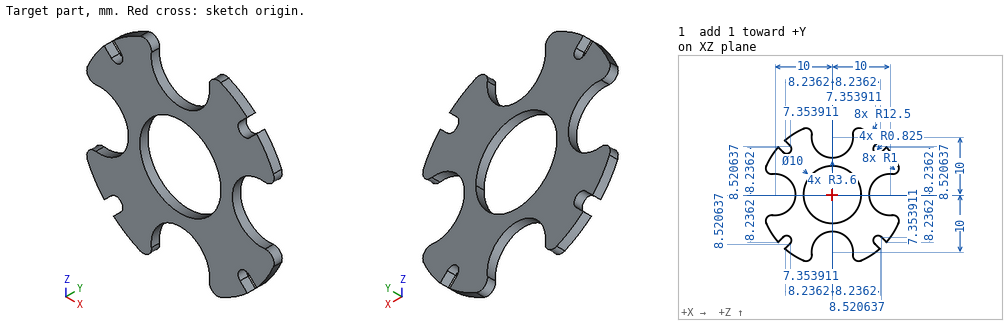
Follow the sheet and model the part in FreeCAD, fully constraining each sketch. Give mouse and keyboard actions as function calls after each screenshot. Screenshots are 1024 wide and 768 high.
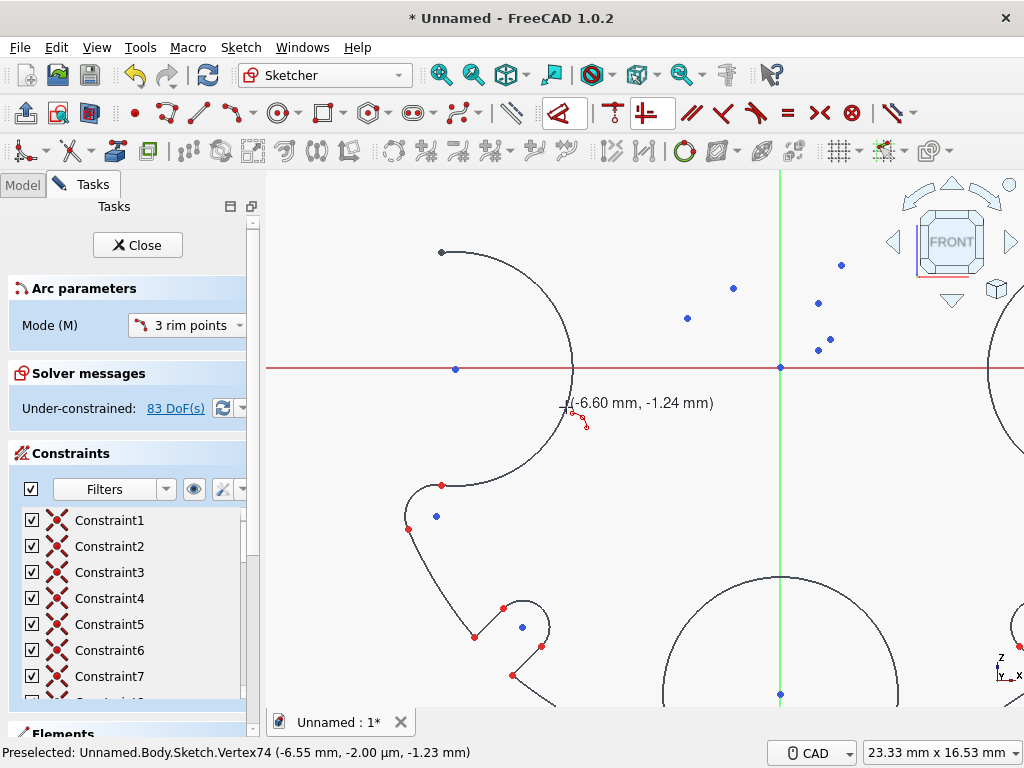
click(441, 253)
click(408, 206)
click(411, 239)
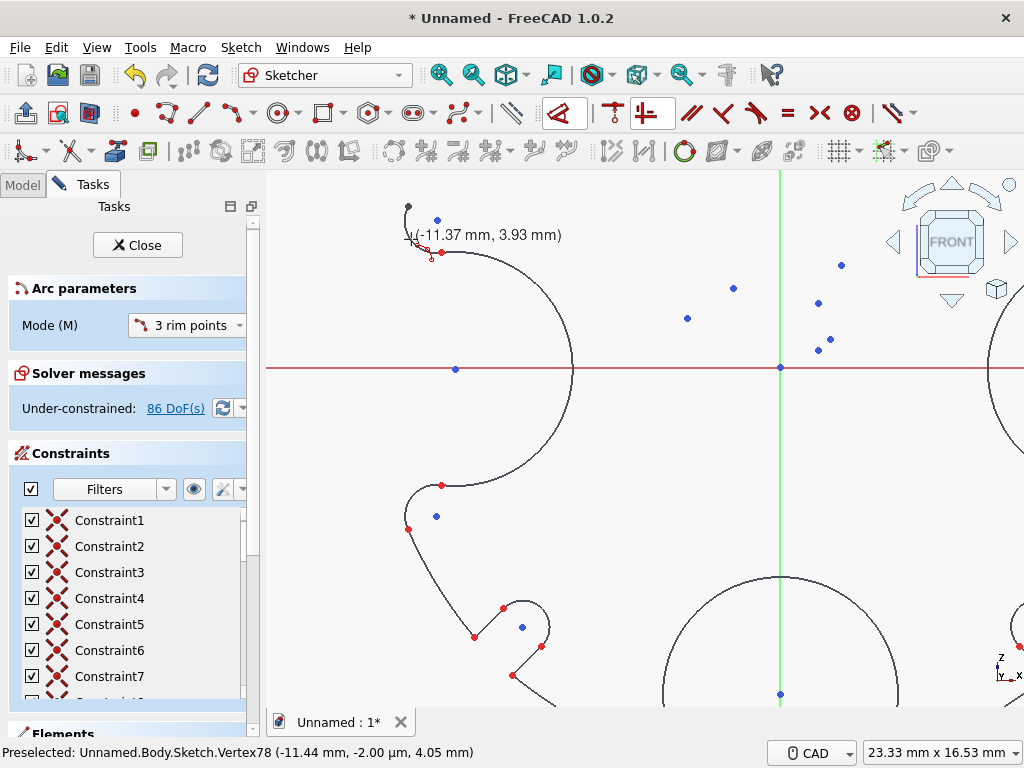
click(408, 207)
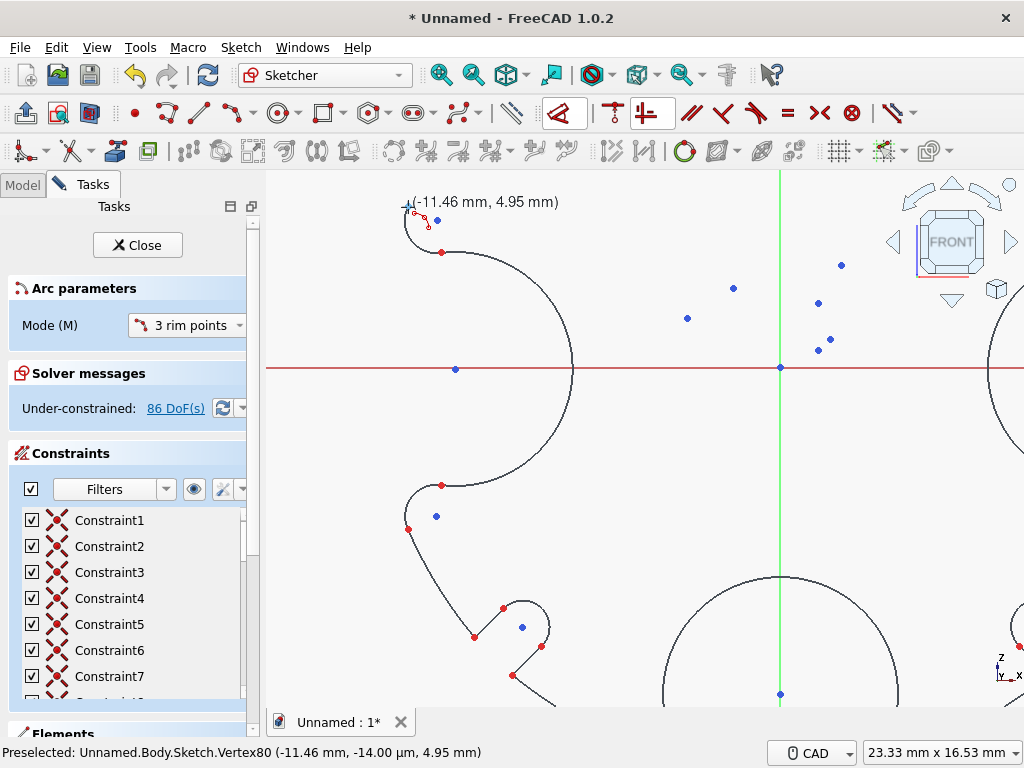
scroll(410, 496, down, 4)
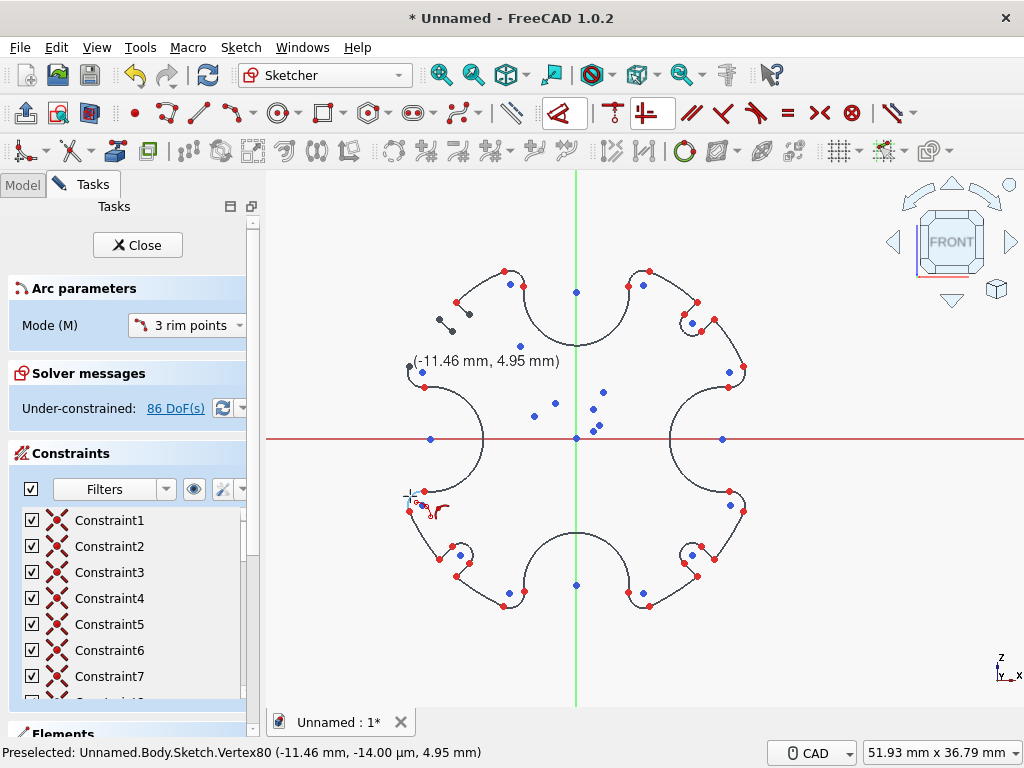
scroll(439, 318, up, 3)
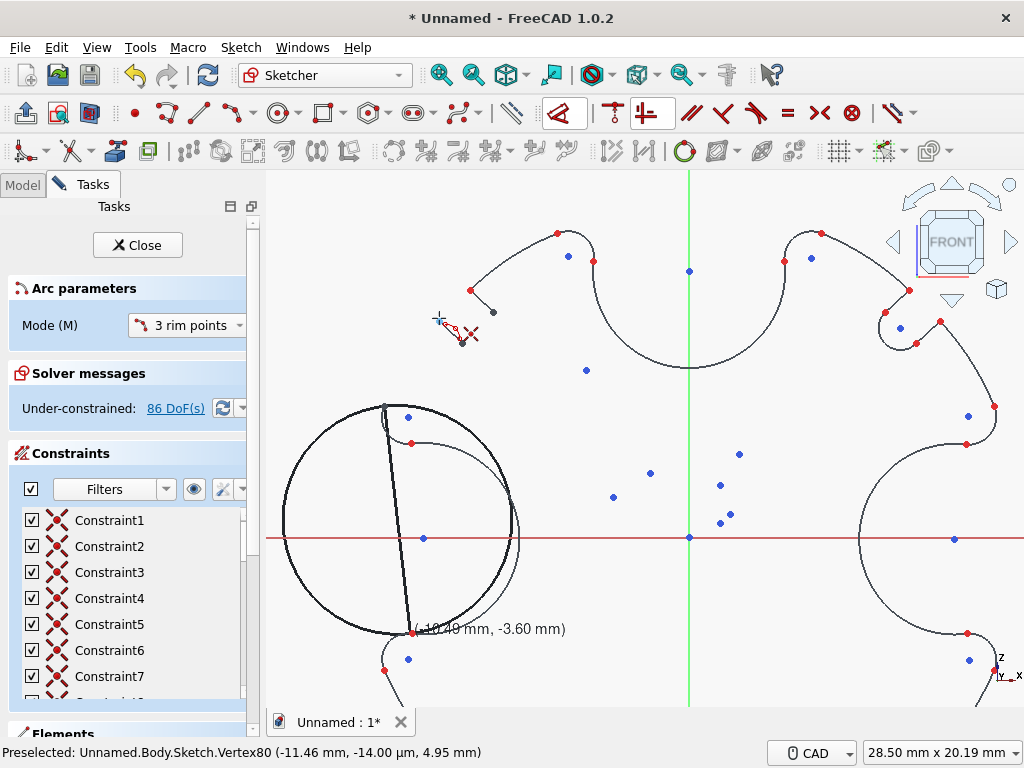
click(439, 321)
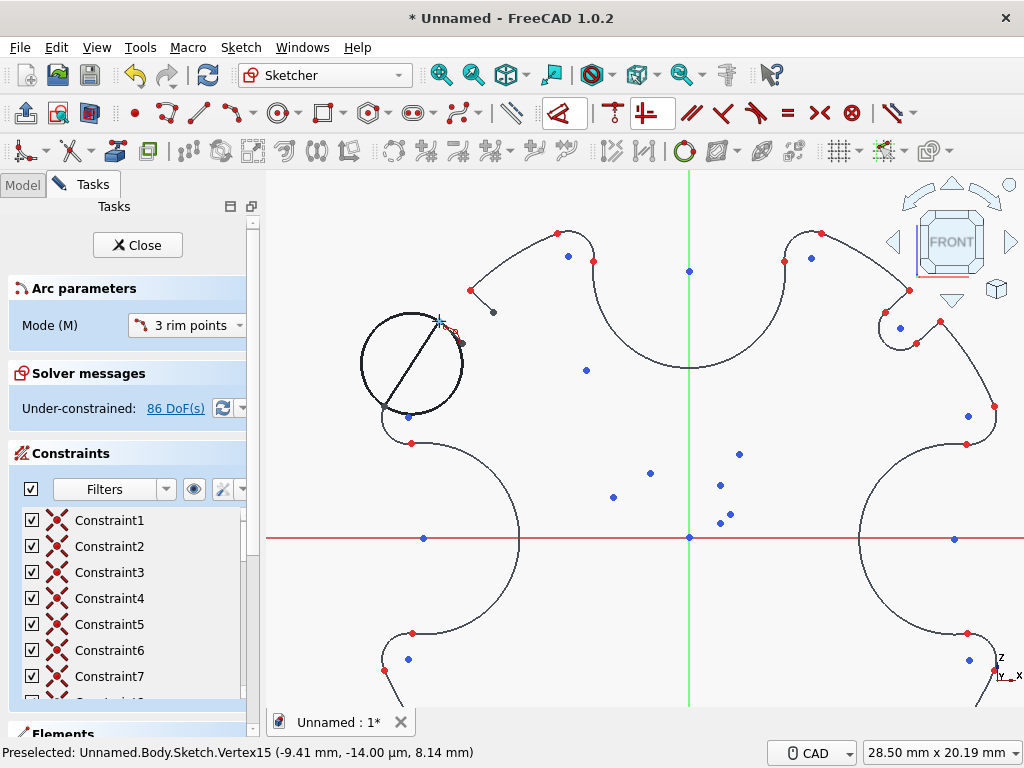
scroll(408, 360, up, 7)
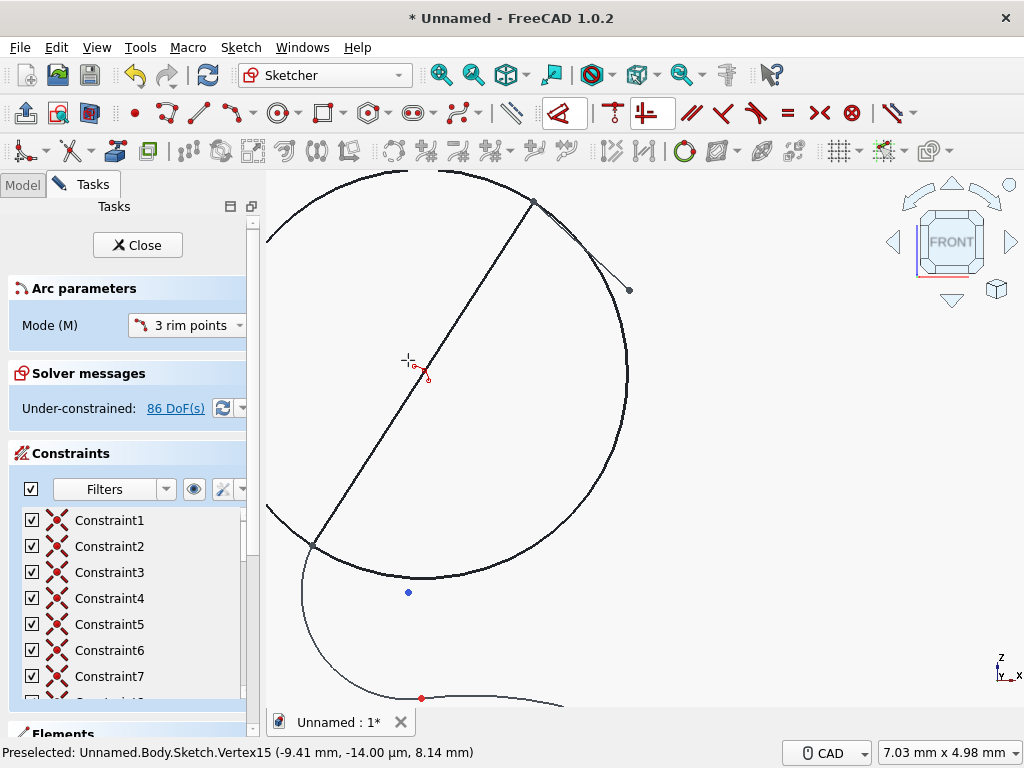
click(409, 359)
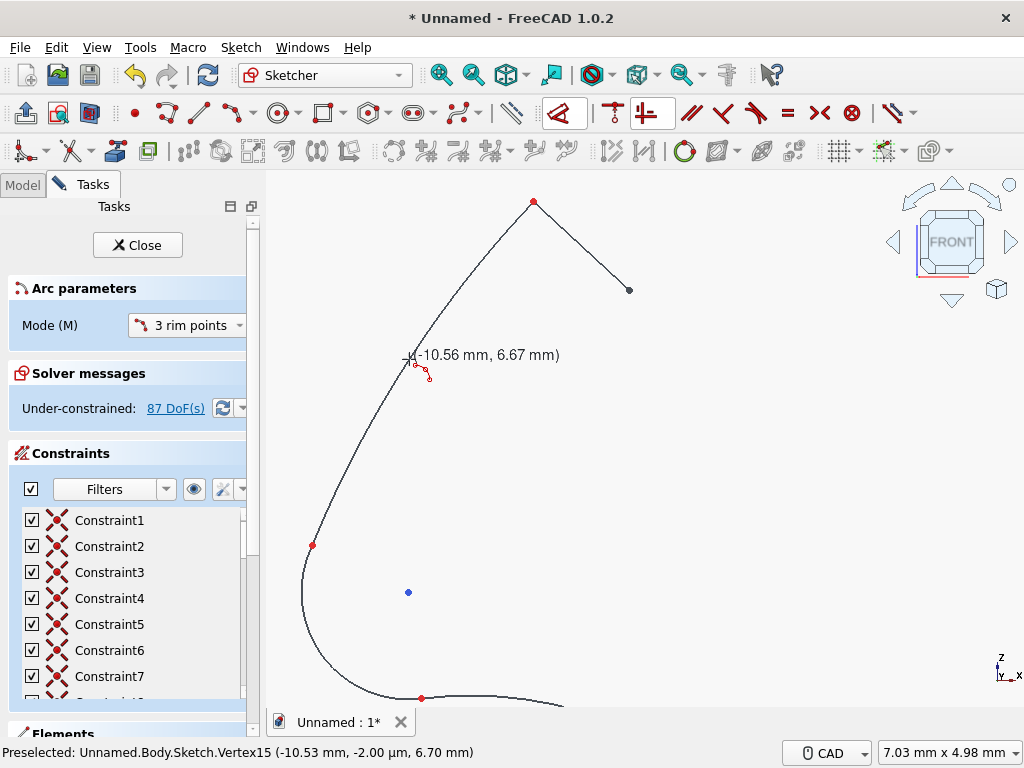
scroll(424, 338, down, 10)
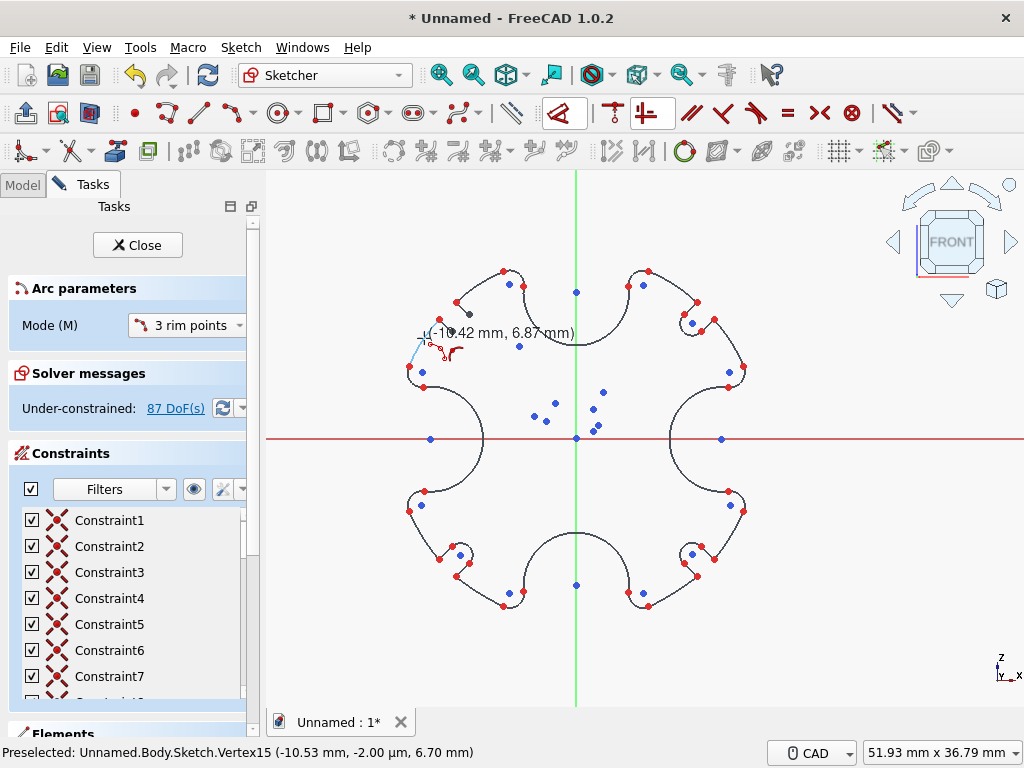
scroll(452, 331, up, 3)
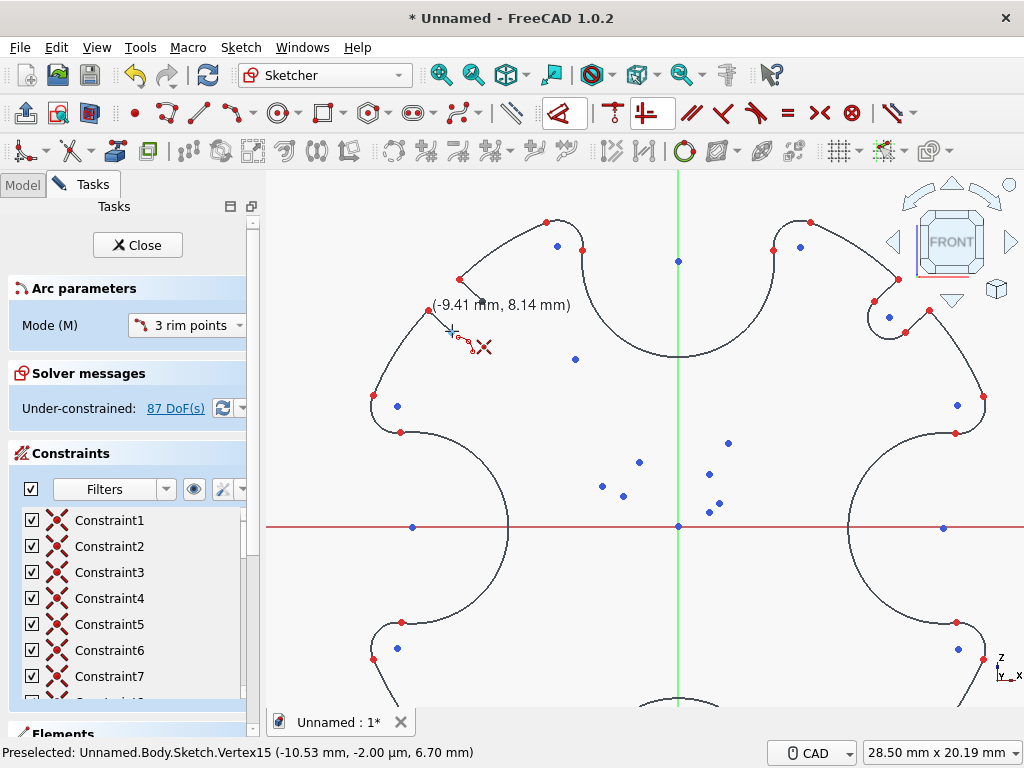
click(452, 332)
click(483, 301)
click(483, 331)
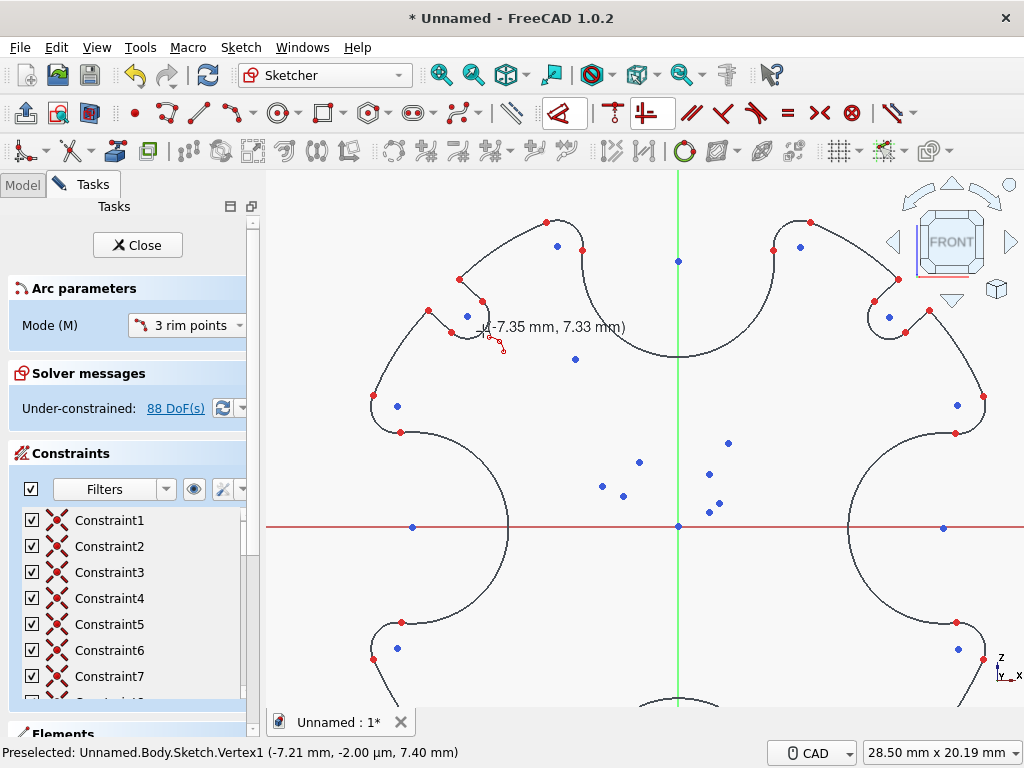
click(278, 114)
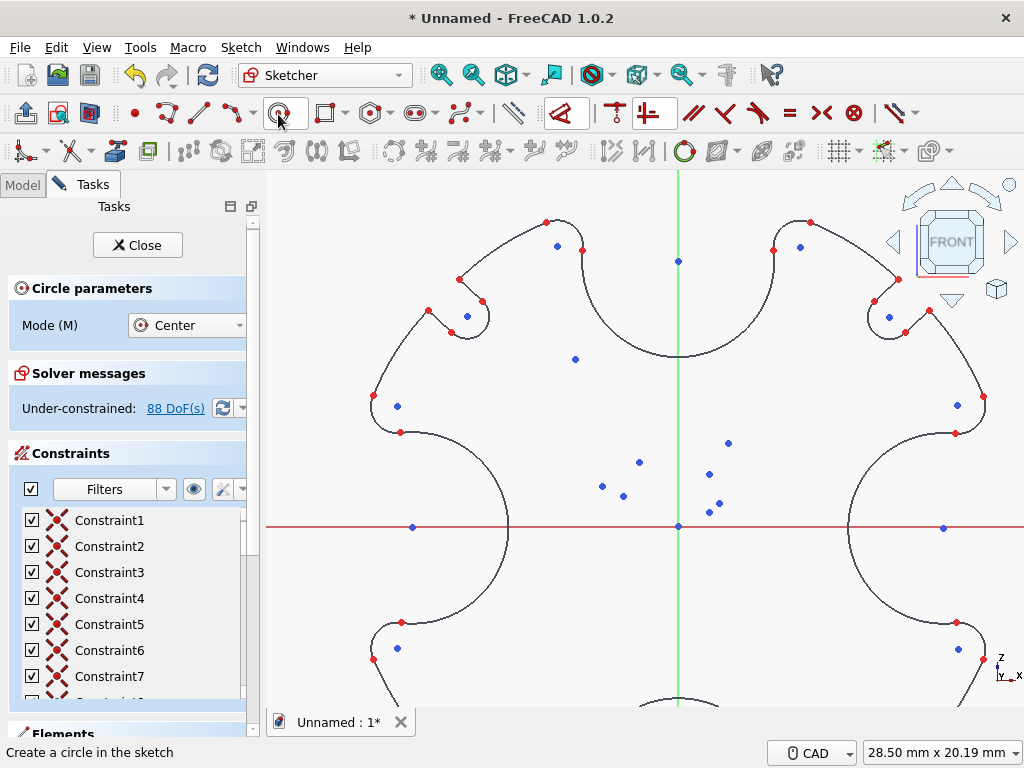
click(678, 527)
click(772, 433)
key(Escape)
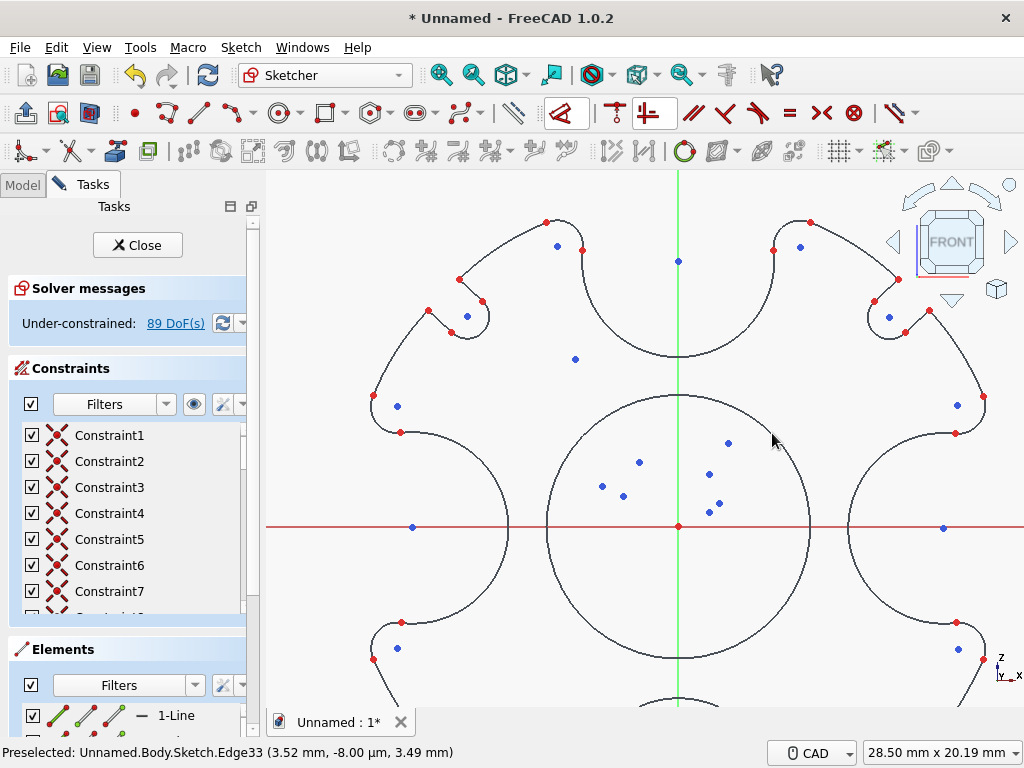
scroll(476, 295, up, 2)